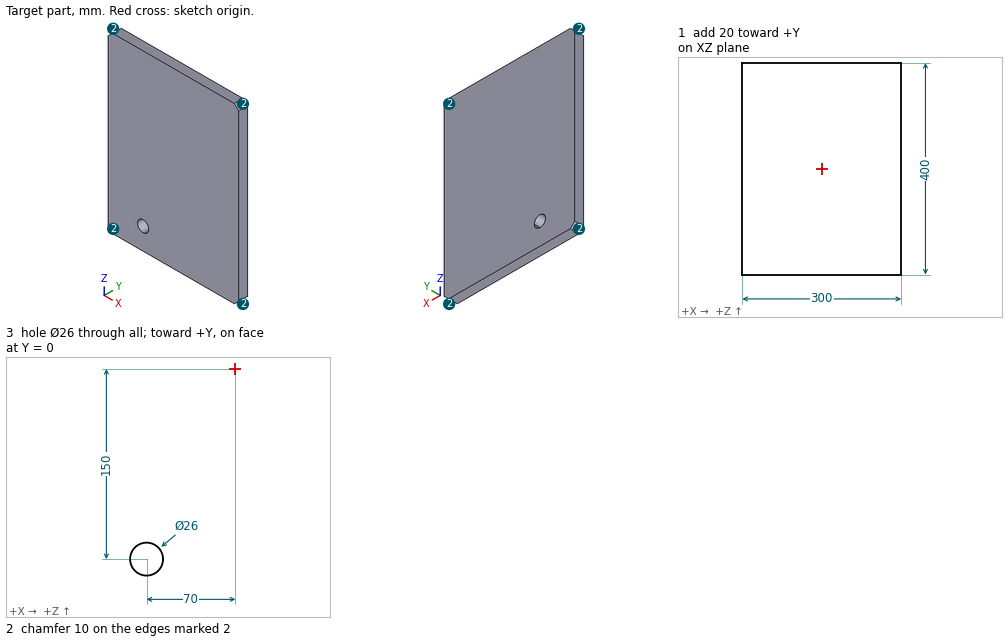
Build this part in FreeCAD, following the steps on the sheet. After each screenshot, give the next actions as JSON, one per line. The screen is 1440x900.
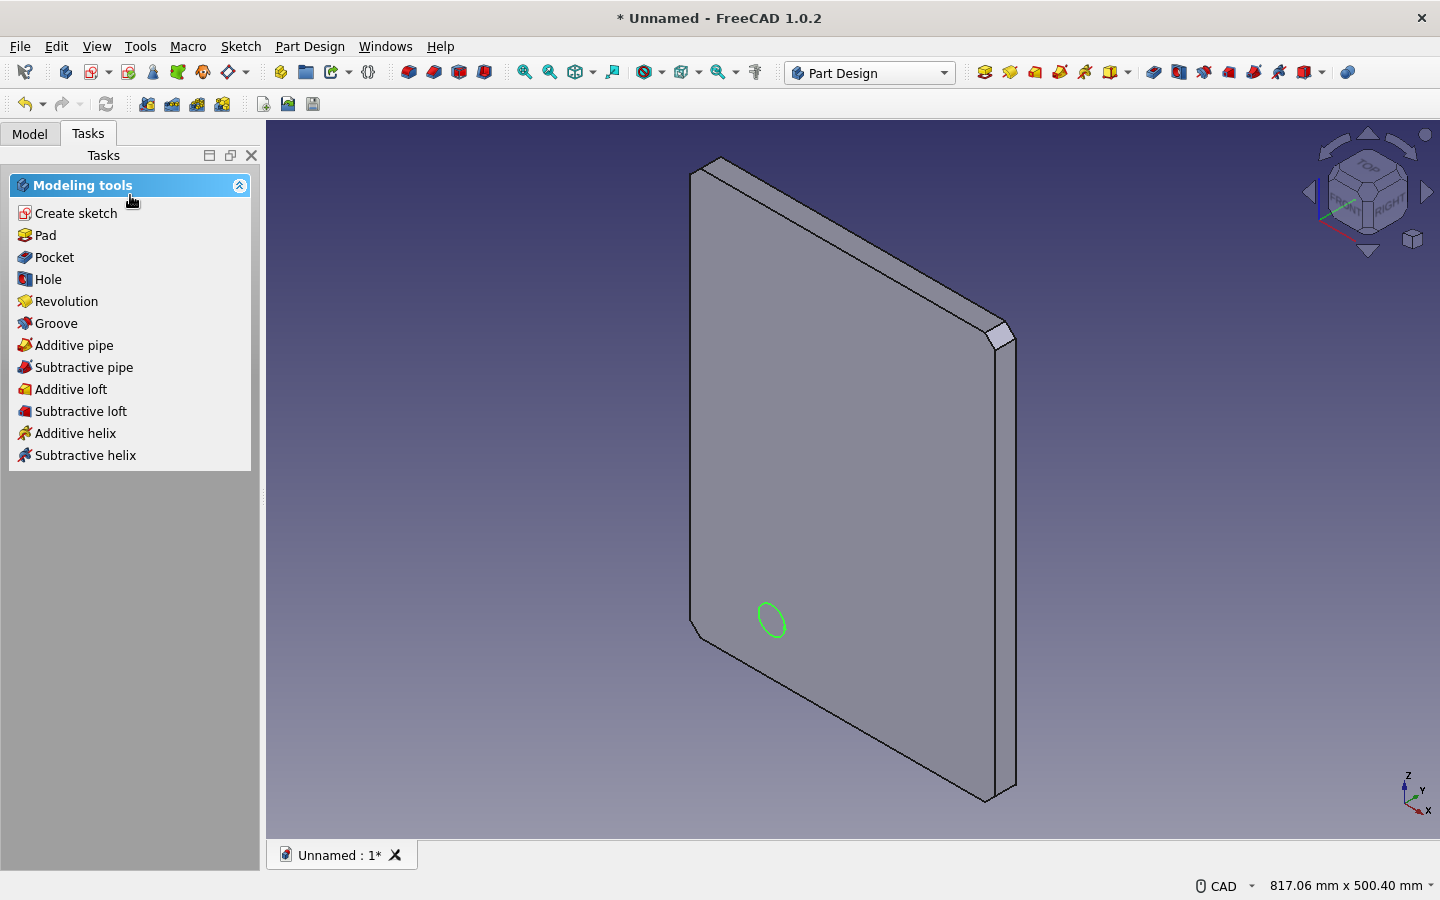
{"action": "left_click", "coordinate": [1179, 72]}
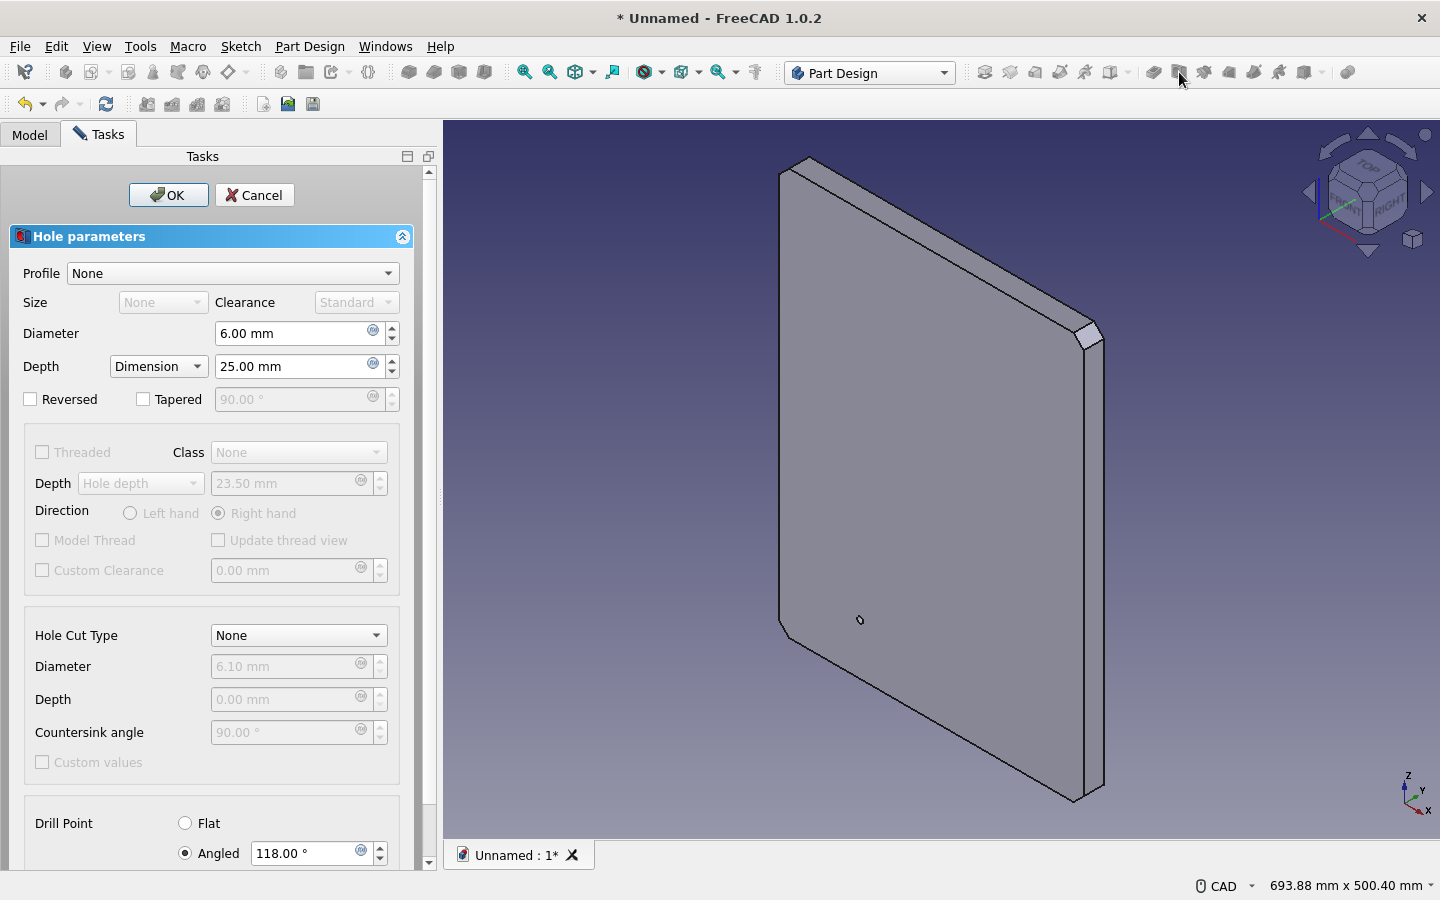
{"action": "triple_click", "coordinate": [300, 334]}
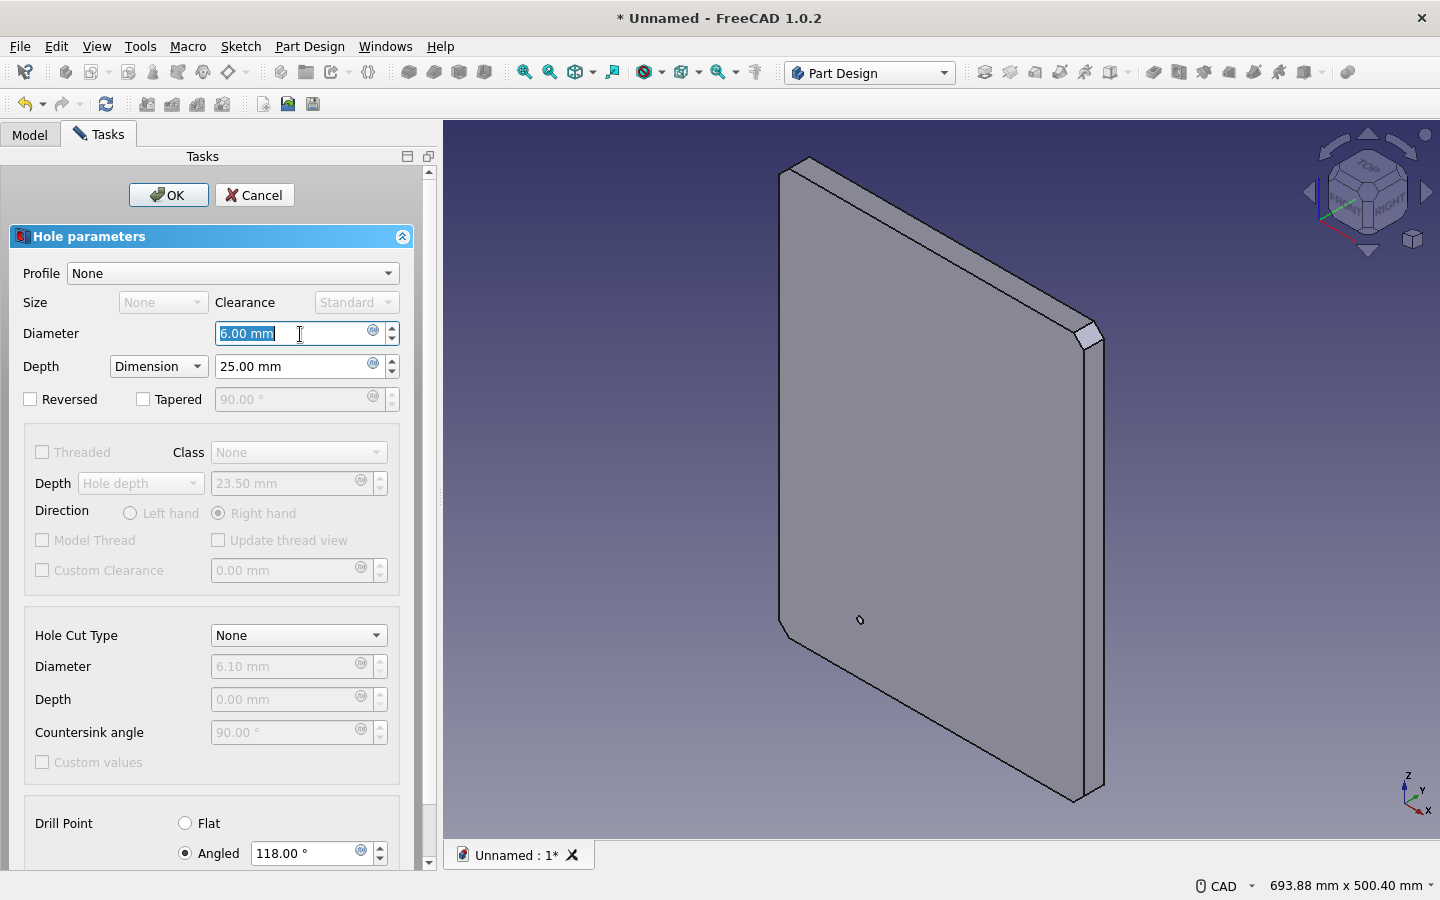
{"action": "type", "text": "26"}
{"action": "key", "text": "Tab"}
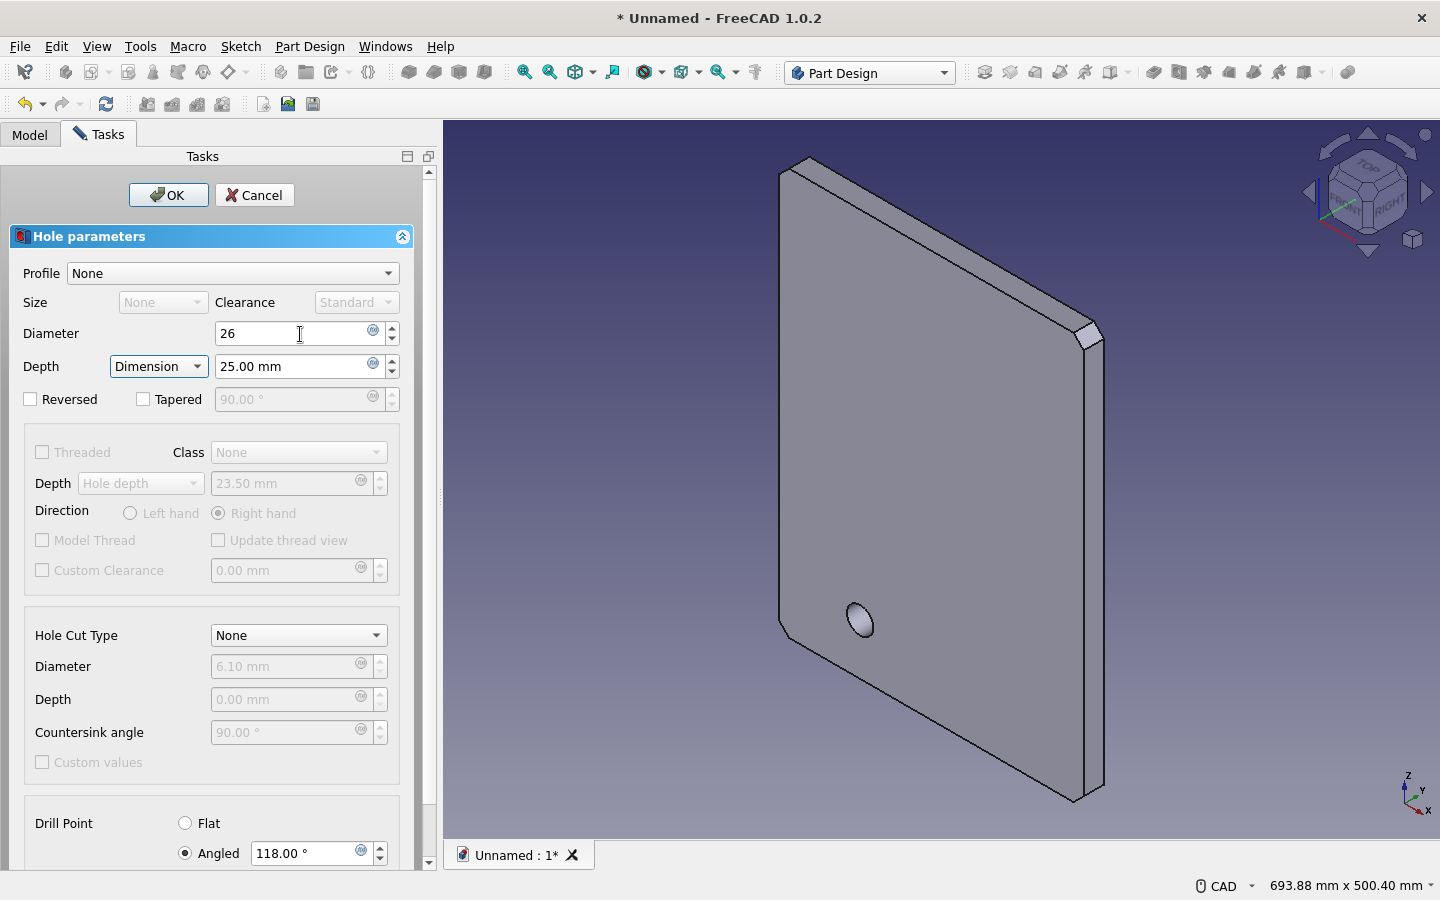
{"action": "left_click", "coordinate": [160, 366]}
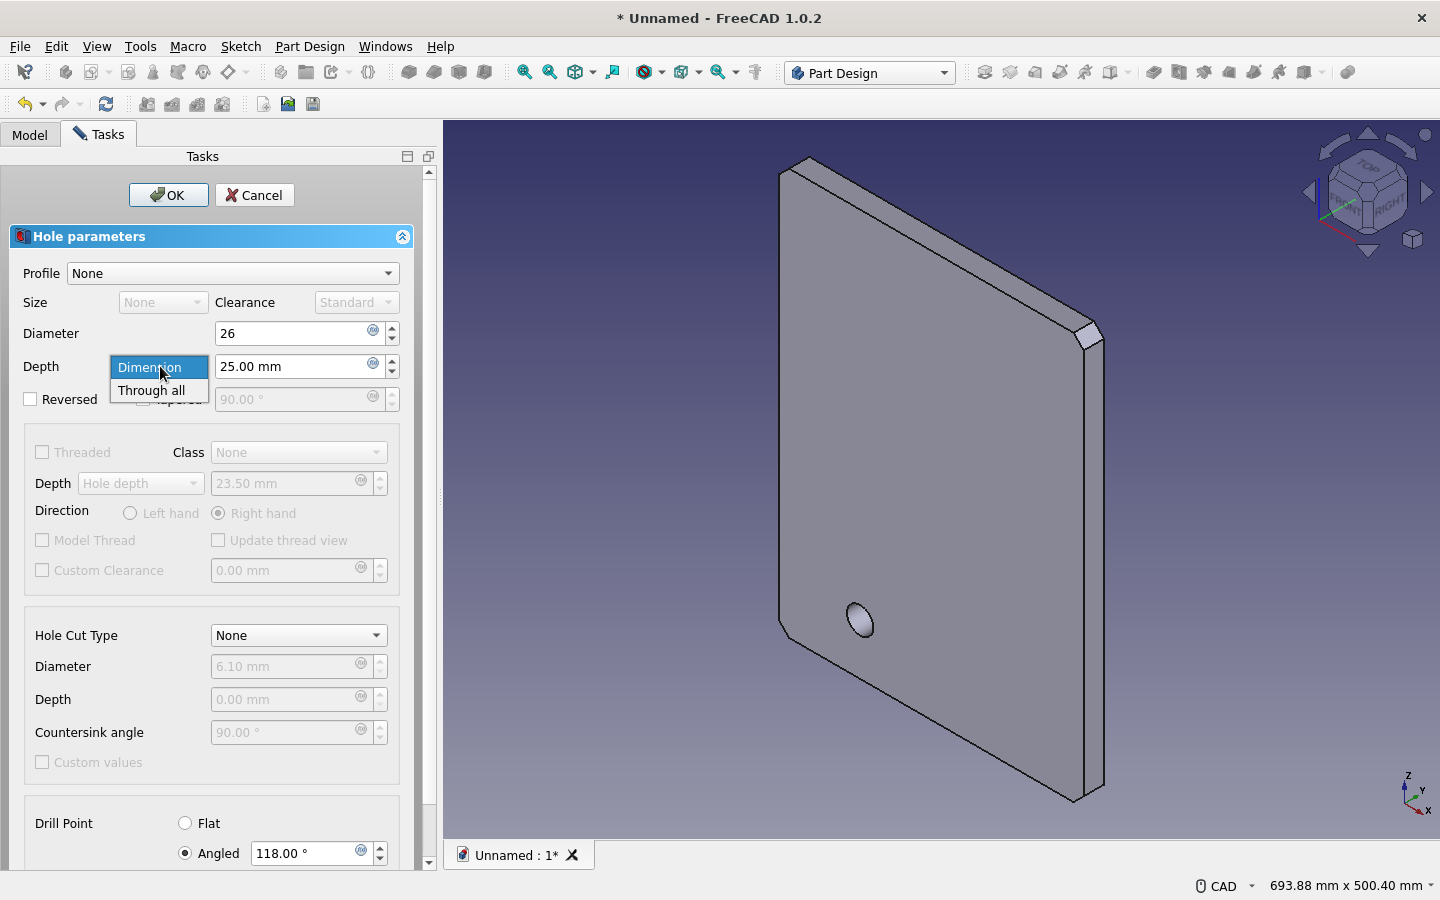
{"action": "left_click", "coordinate": [158, 390]}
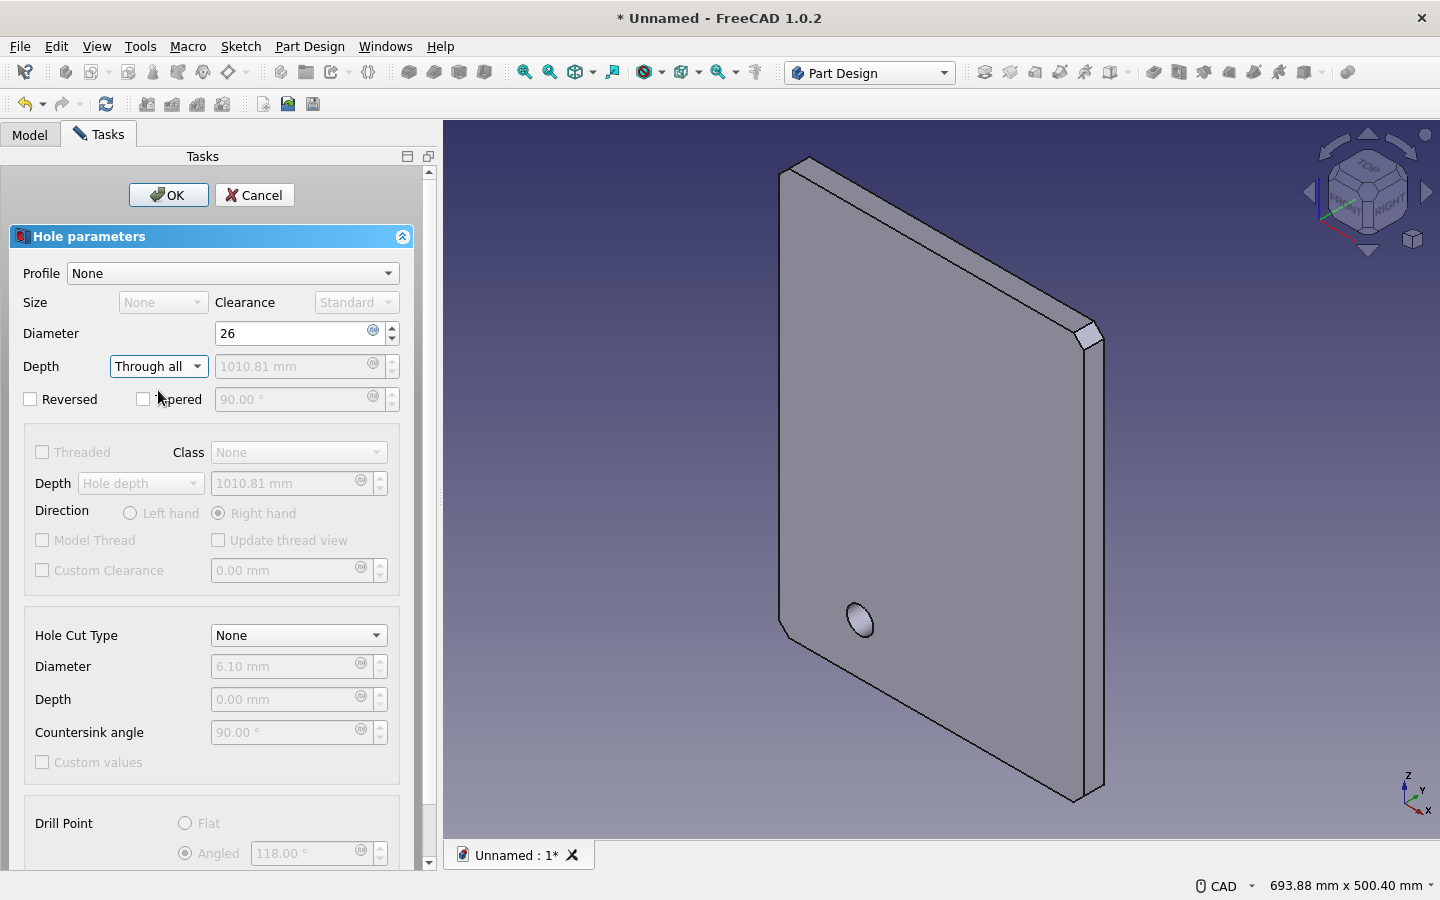
{"action": "left_click", "coordinate": [169, 195]}